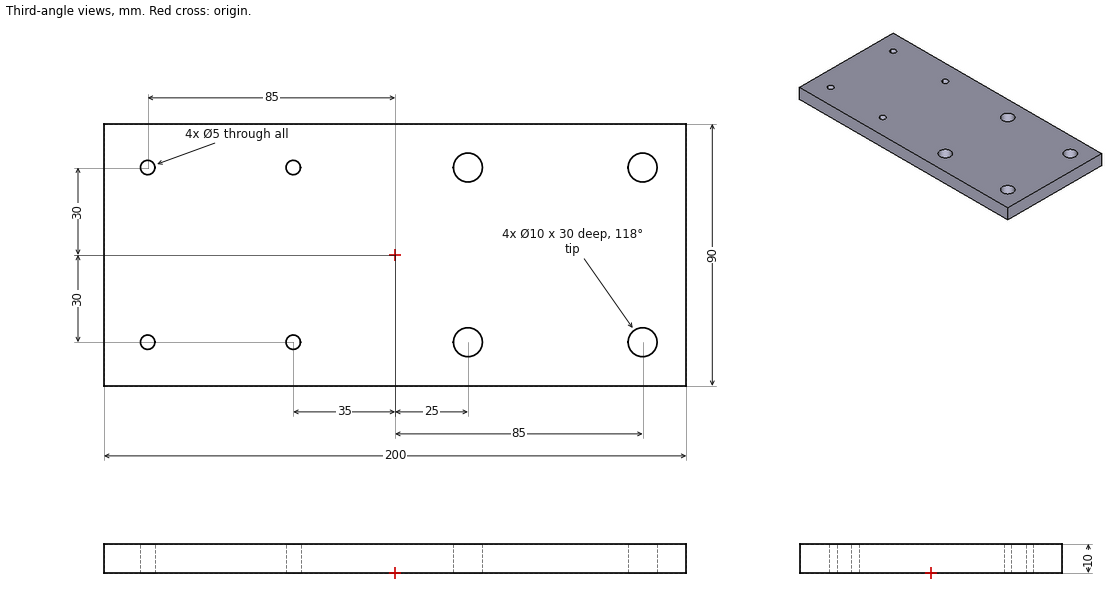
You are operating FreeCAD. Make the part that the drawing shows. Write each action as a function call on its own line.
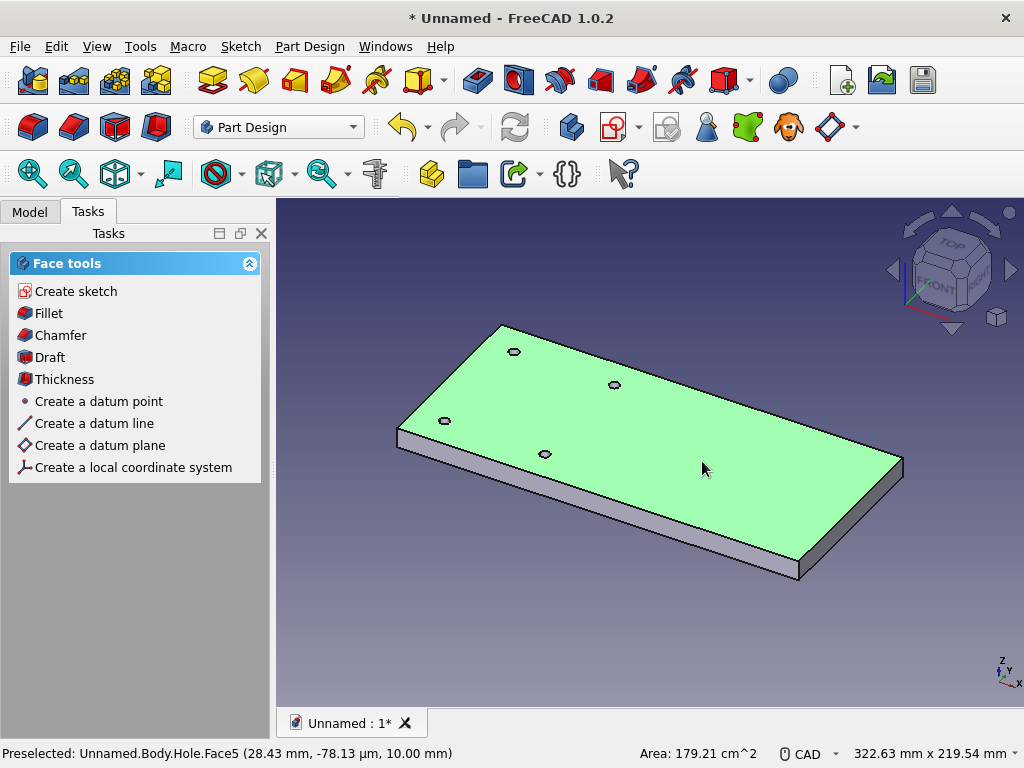
click(612, 128)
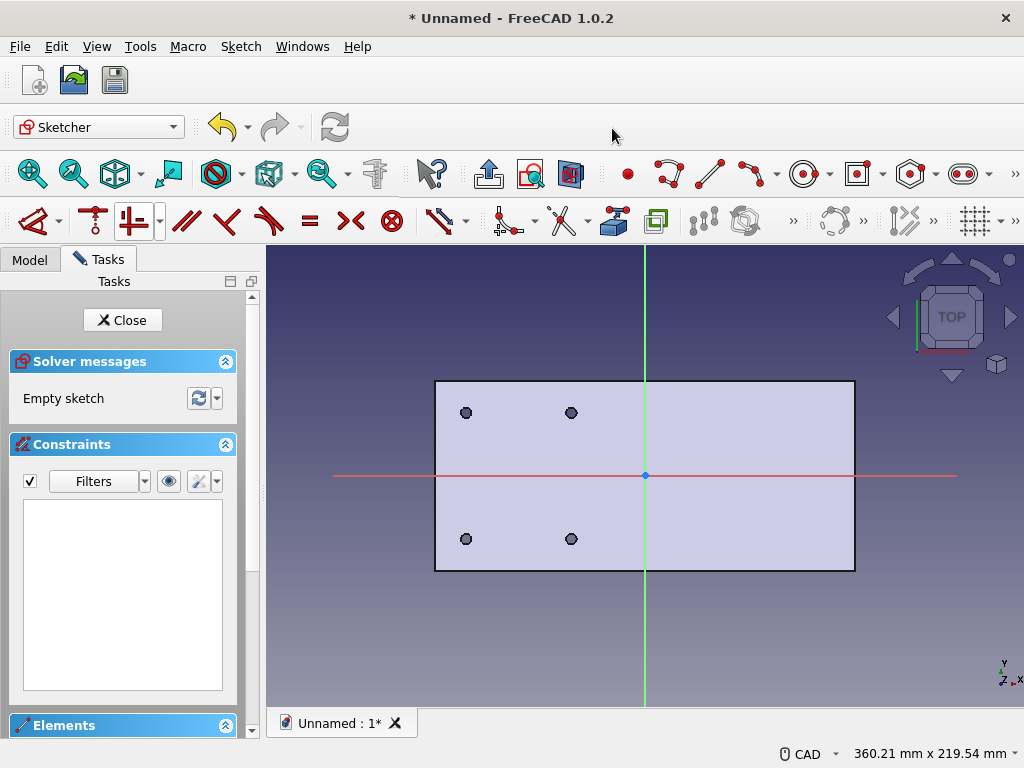
scroll(859, 476, up, 3)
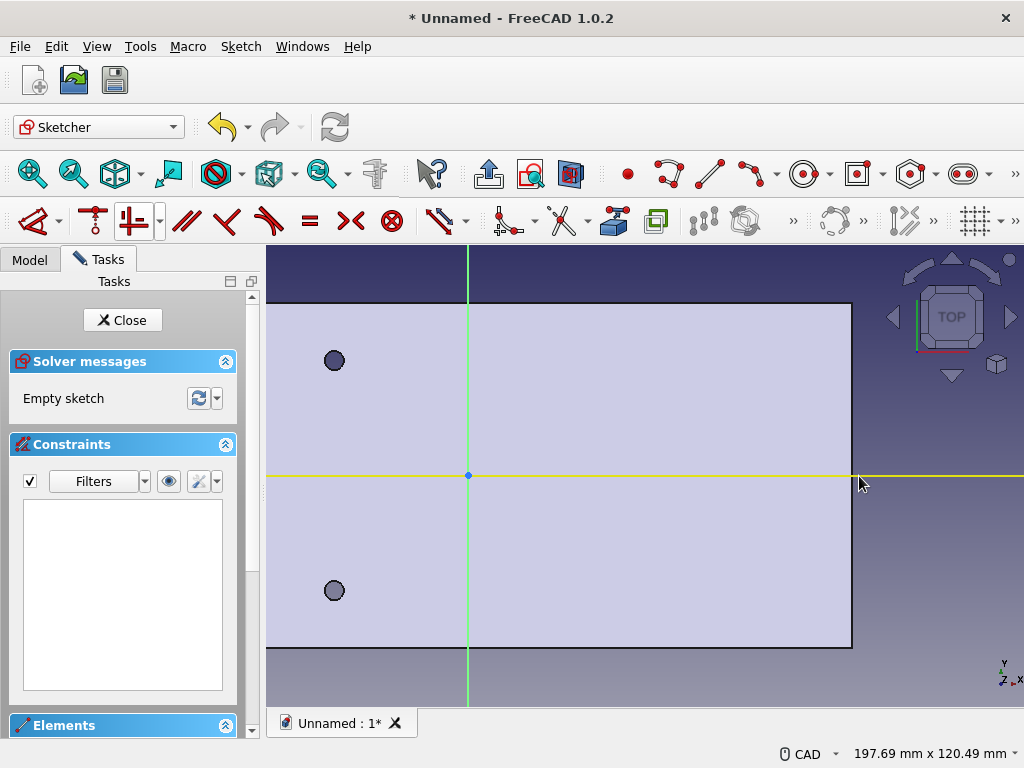
key(g)
key(c)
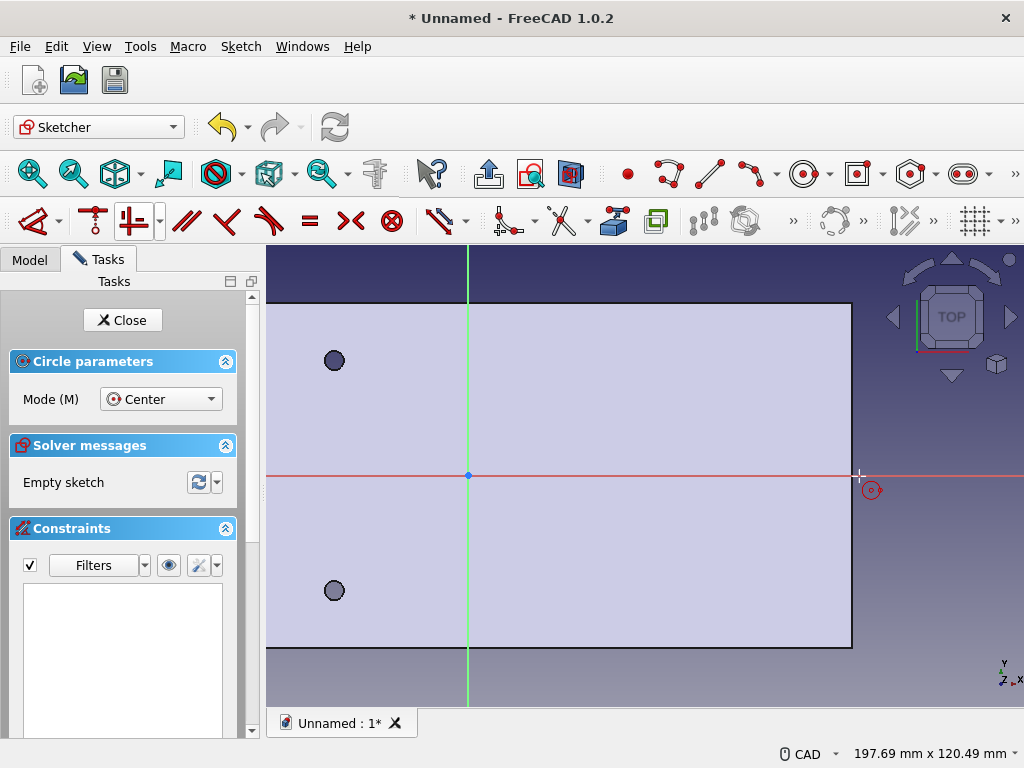
click(794, 591)
move(808, 577)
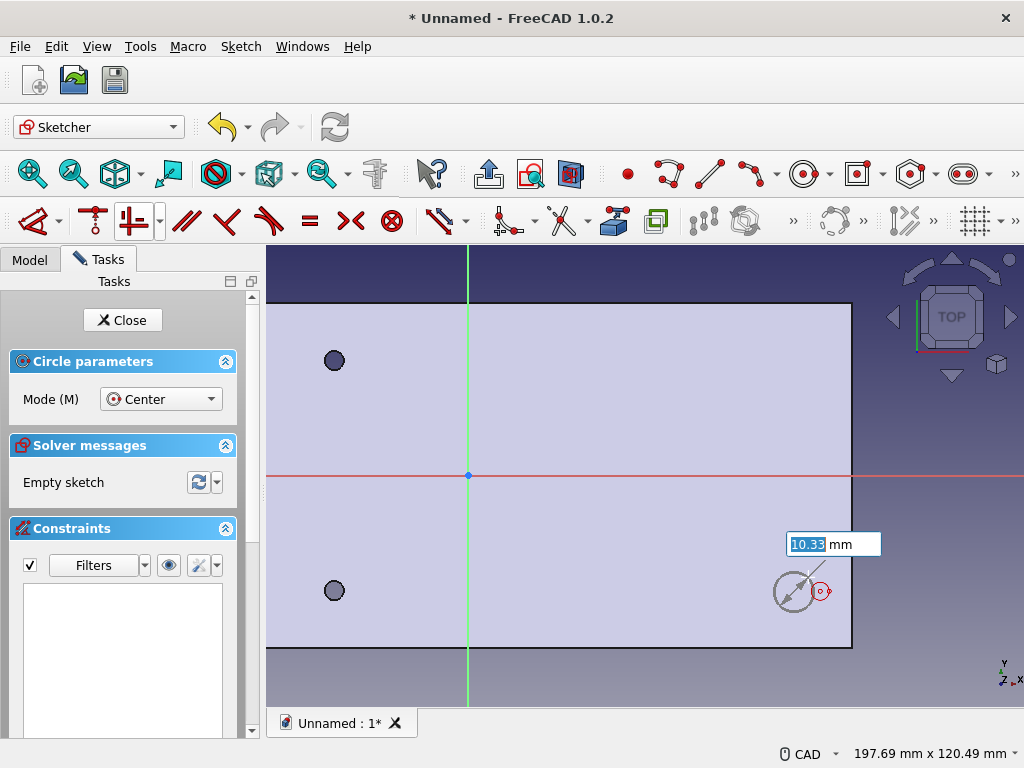
text(10)
key(Return)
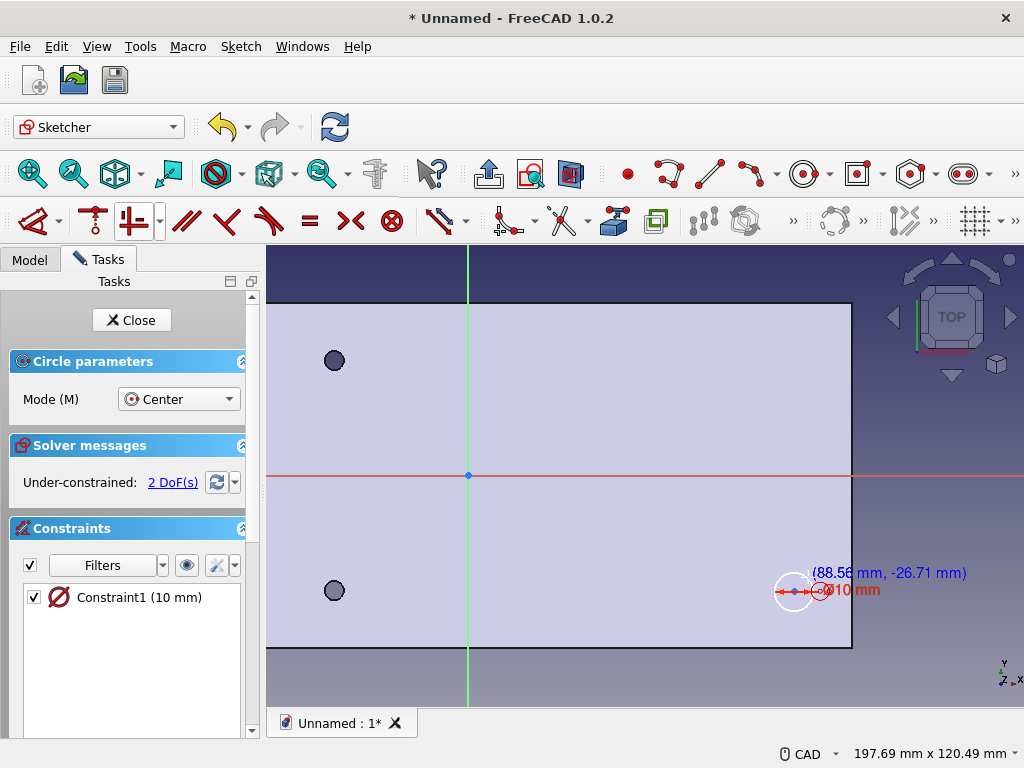
click(794, 361)
move(808, 347)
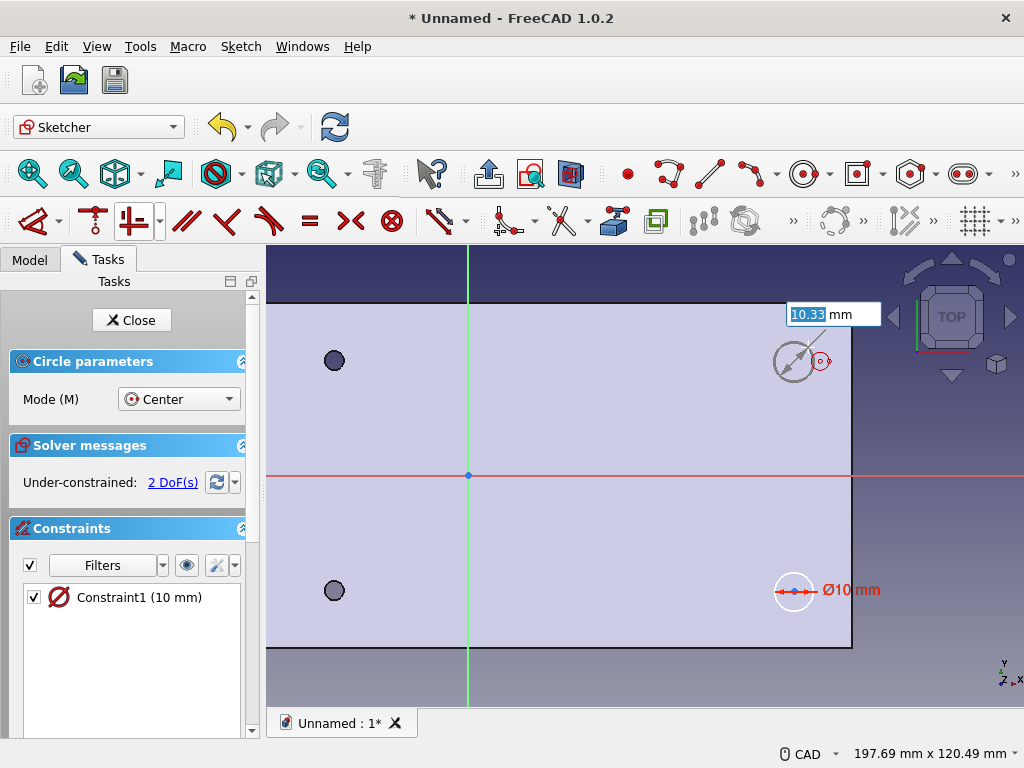
text(10)
key(Return)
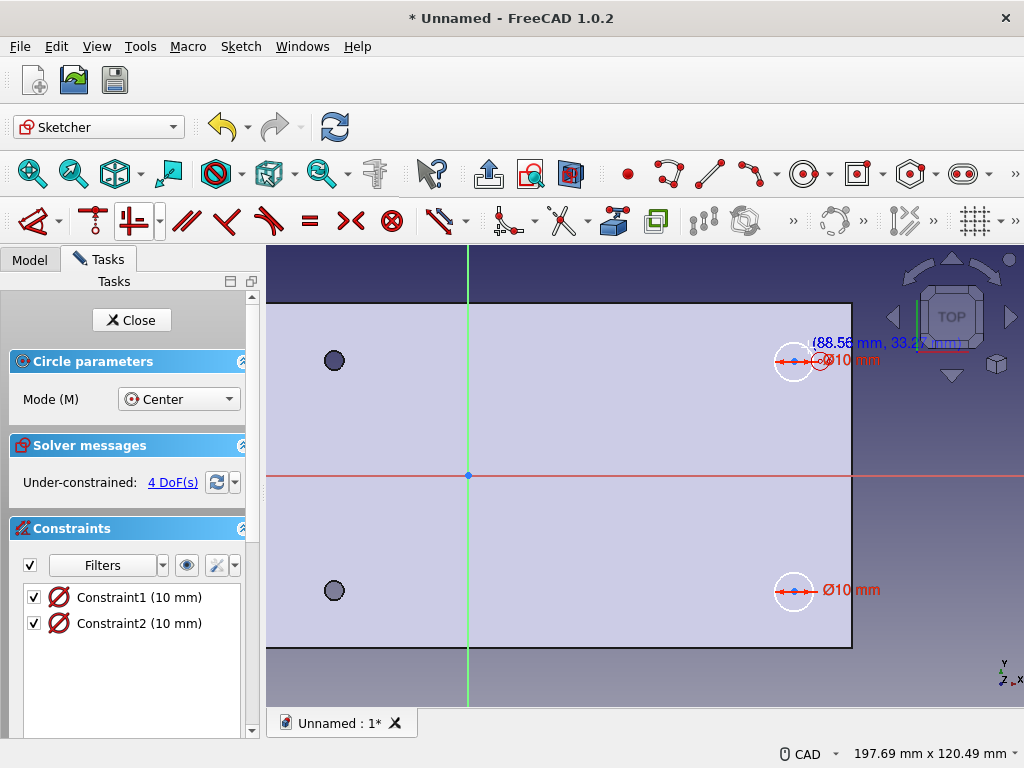
click(564, 591)
move(578, 577)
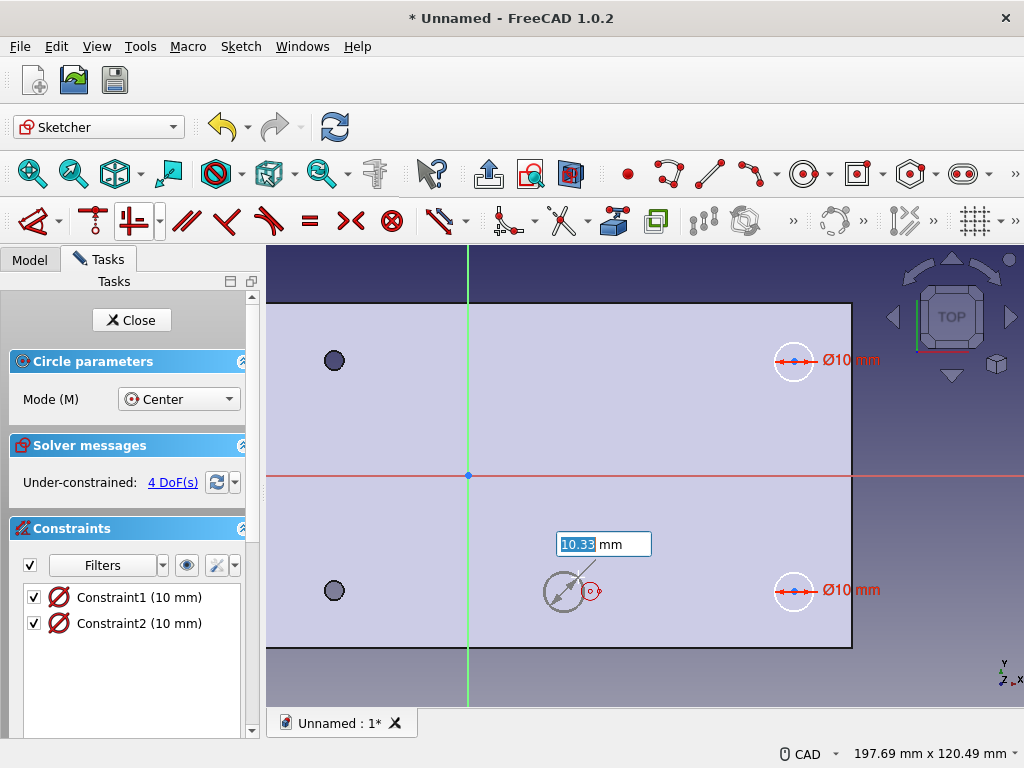
text(10)
key(Return)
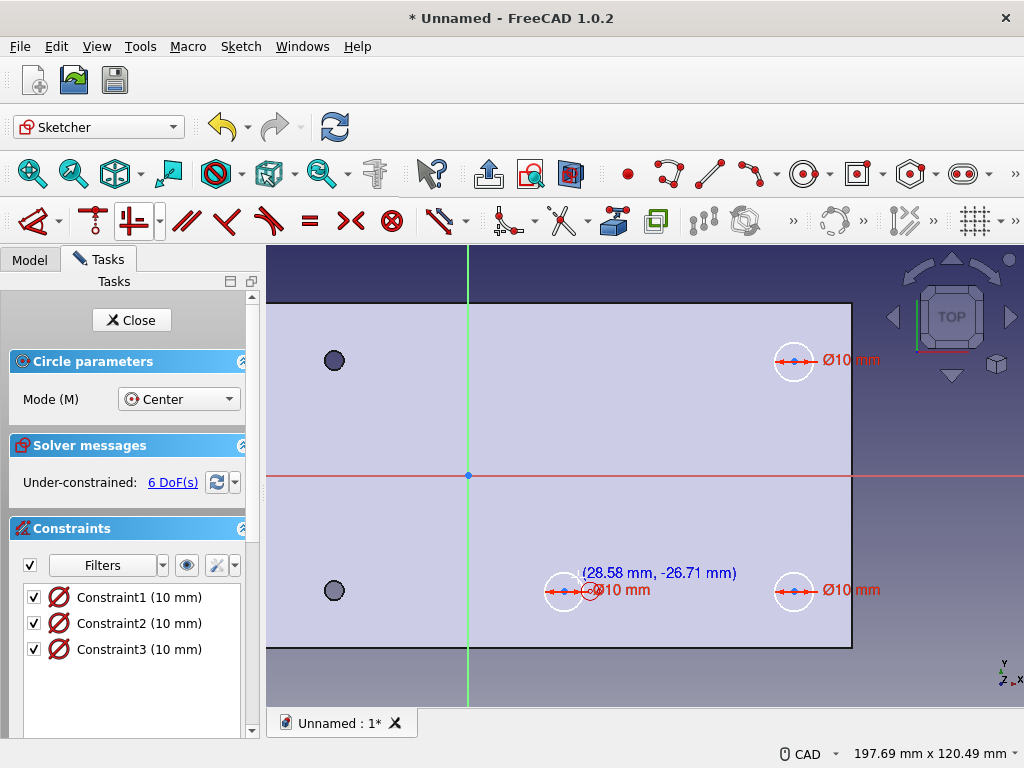
click(564, 361)
move(578, 347)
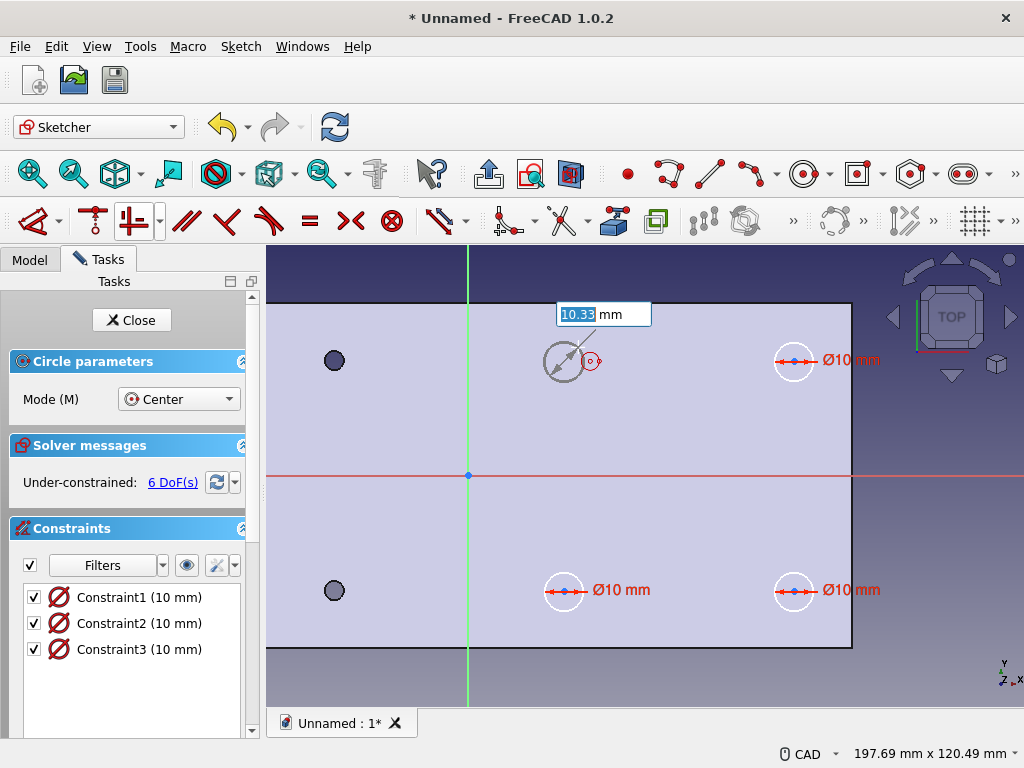
text(10)
key(Return)
key(Escape)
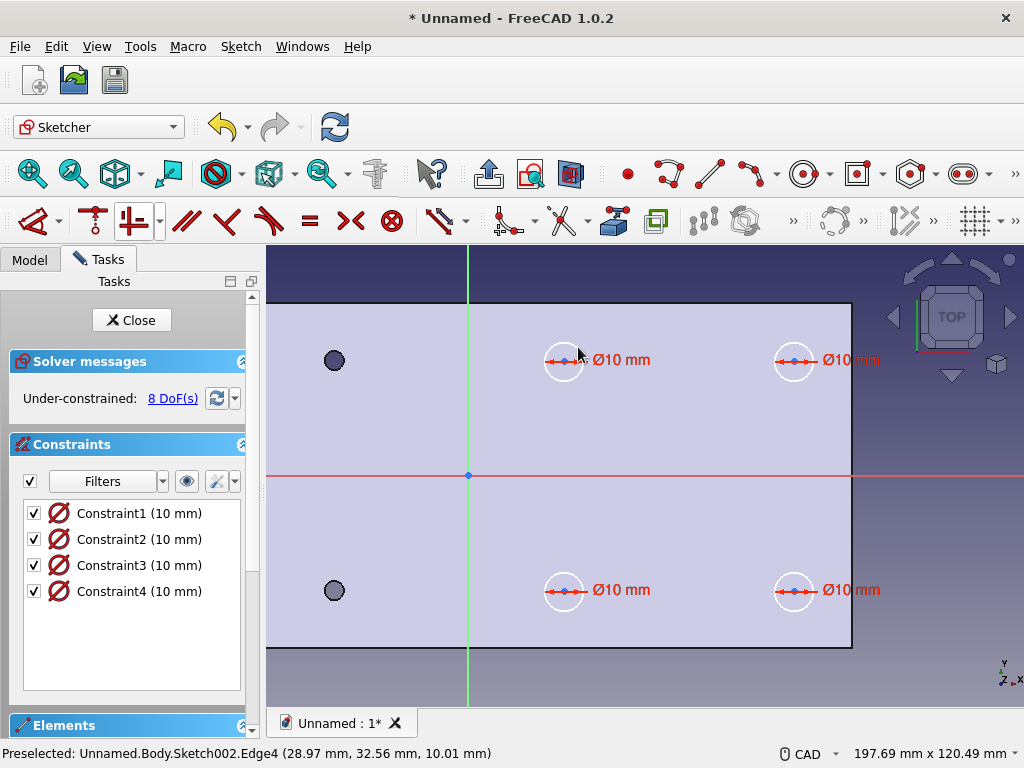
click(794, 592)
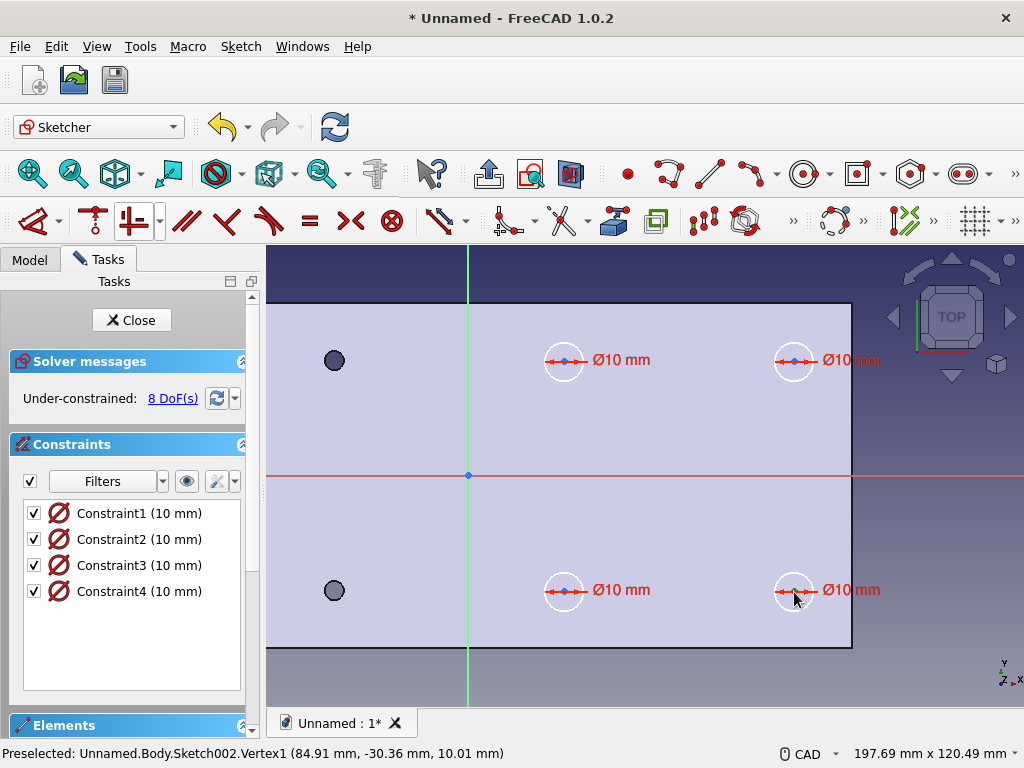
click(794, 362)